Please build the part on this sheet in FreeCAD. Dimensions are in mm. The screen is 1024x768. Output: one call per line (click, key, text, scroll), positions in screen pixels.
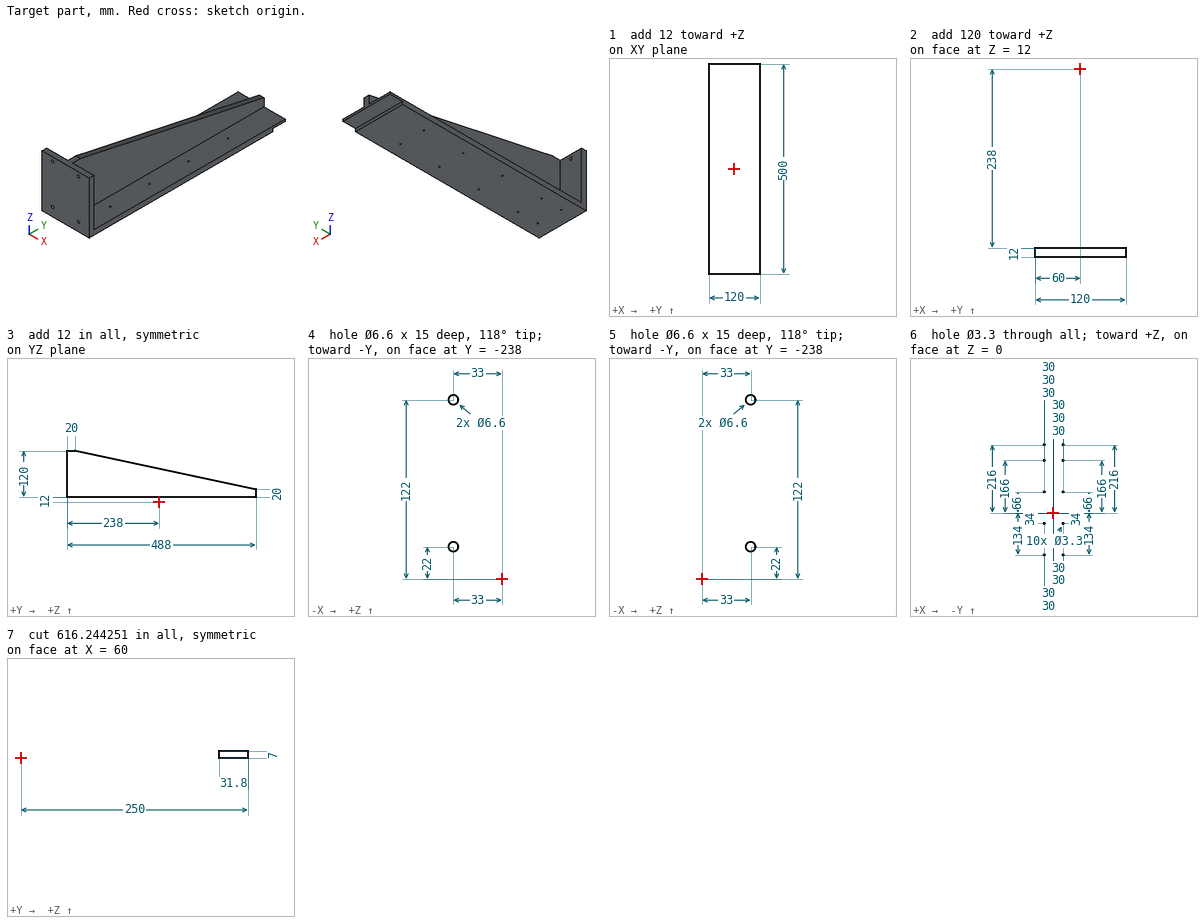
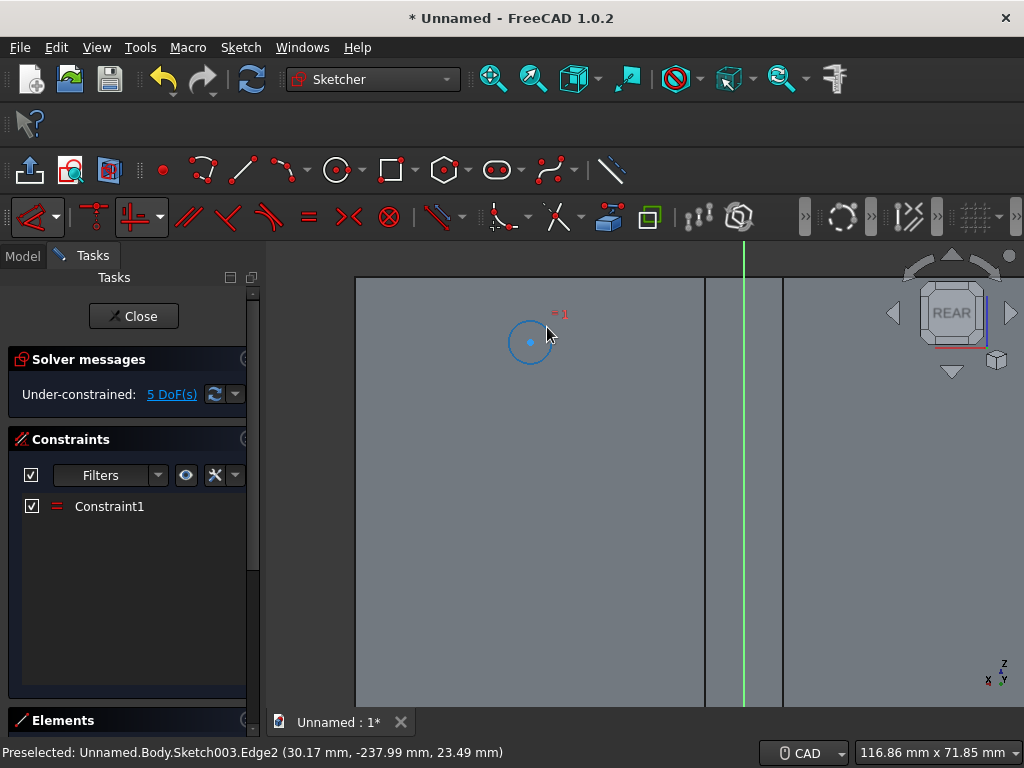
click(545, 327)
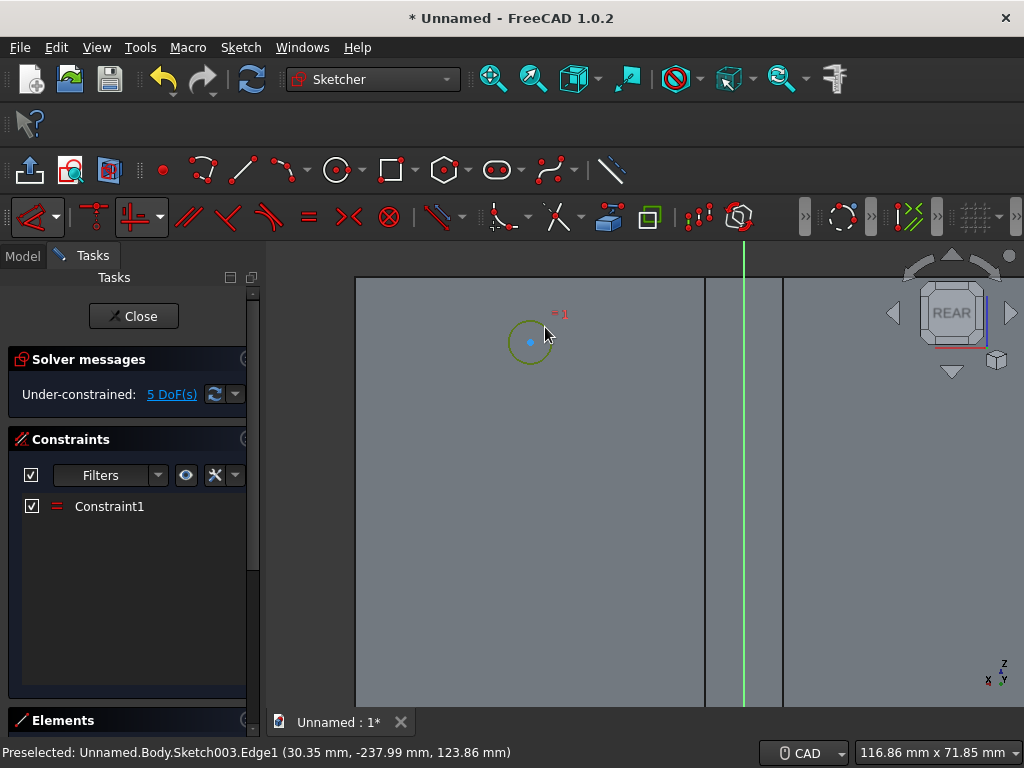
key(k)
key(o)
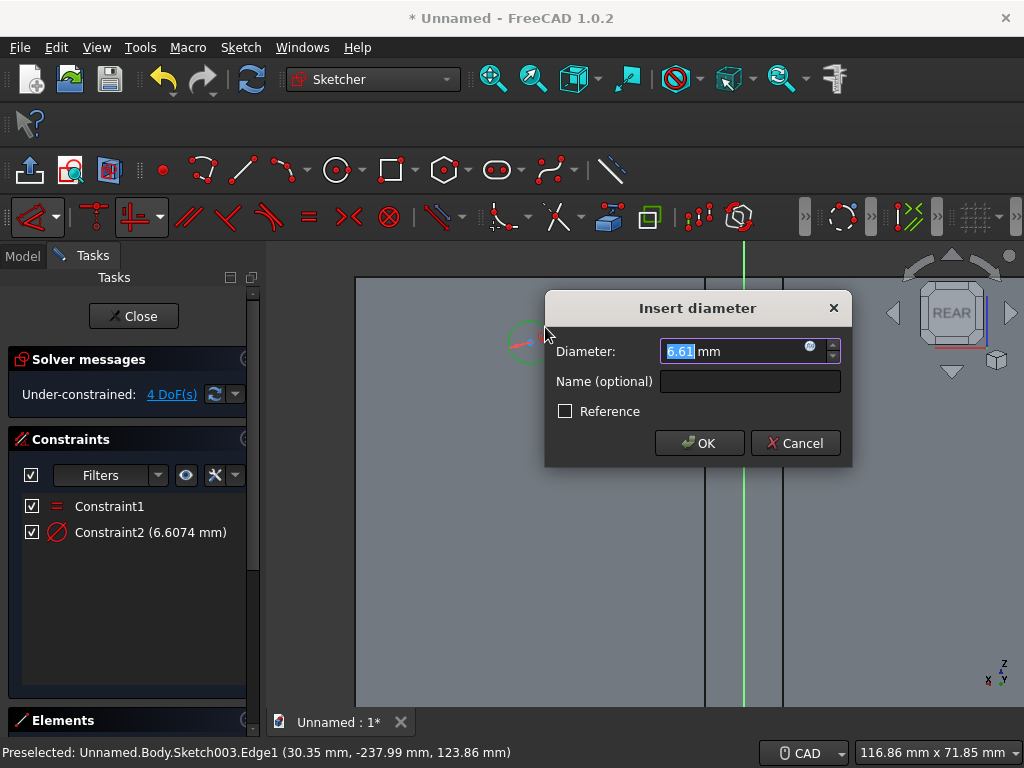
text(6.6)
key(Return)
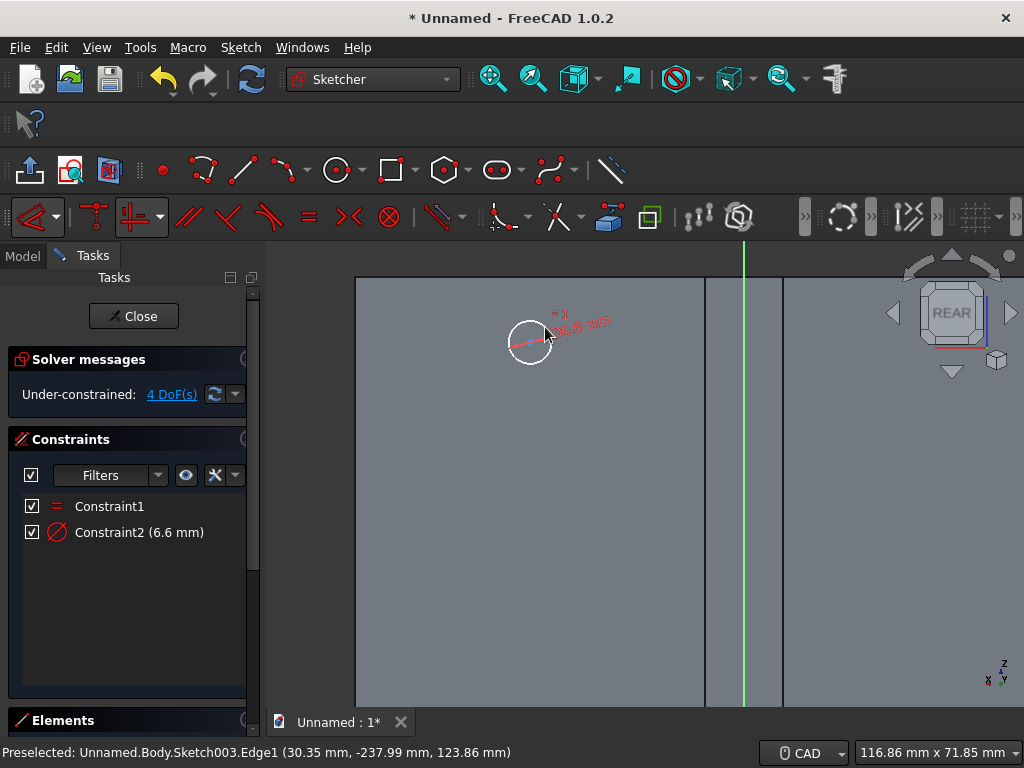
click(530, 342)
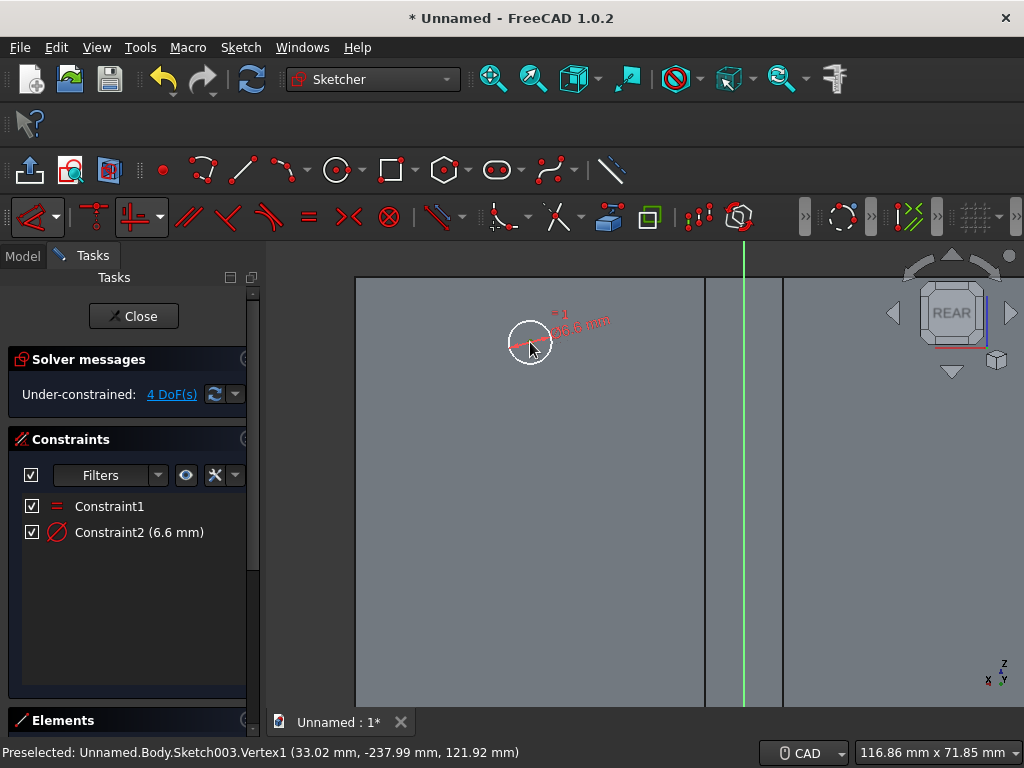
key(l)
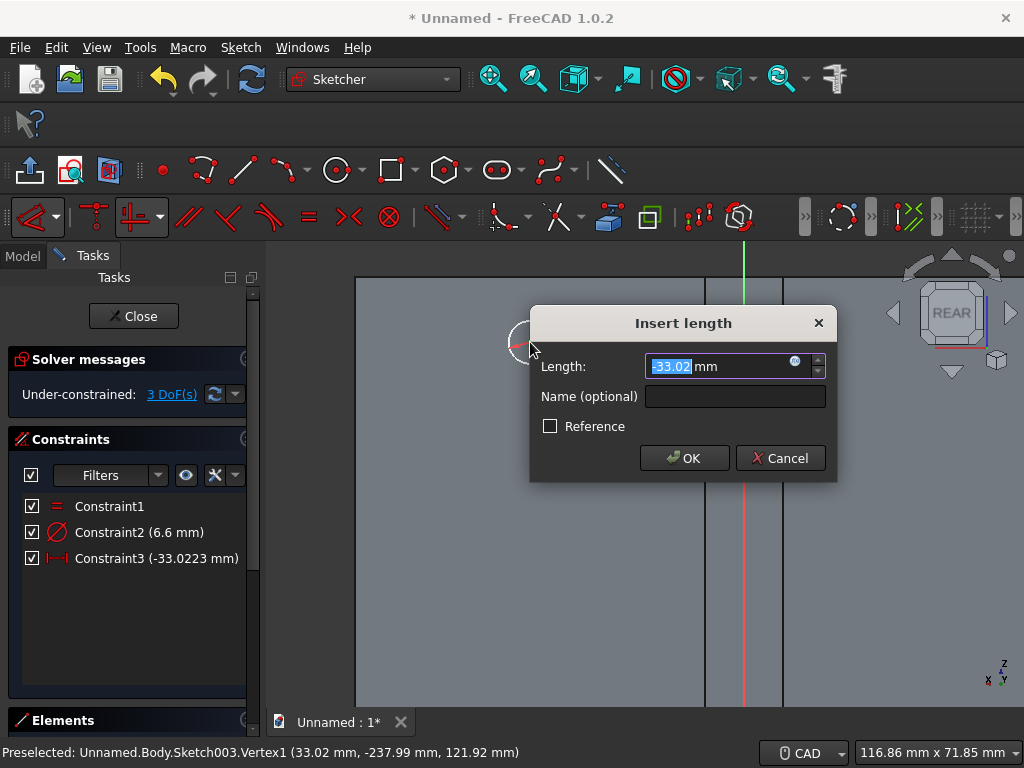
text(-33)
key(Return)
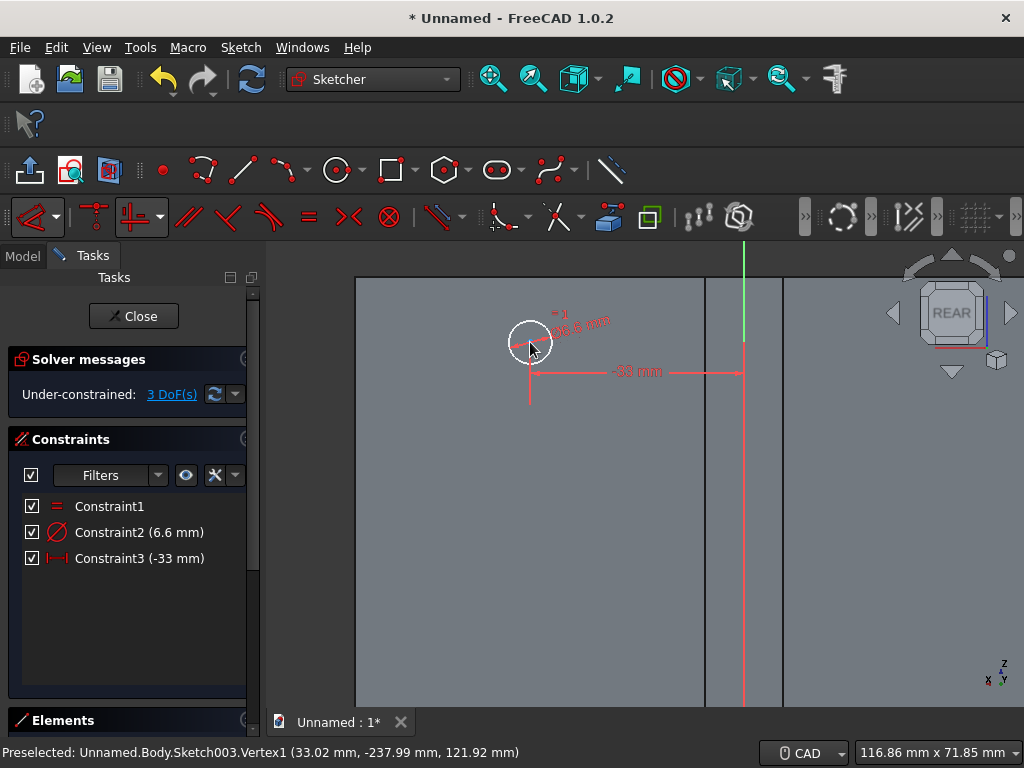
scroll(547, 327, down, 5)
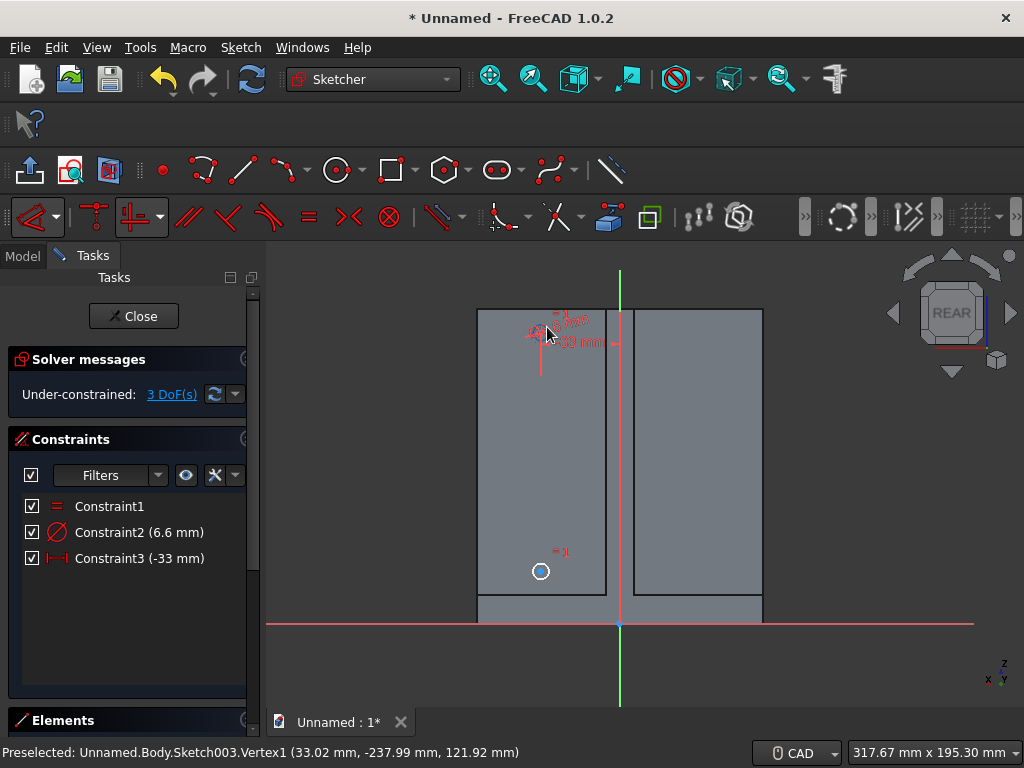
click(541, 571)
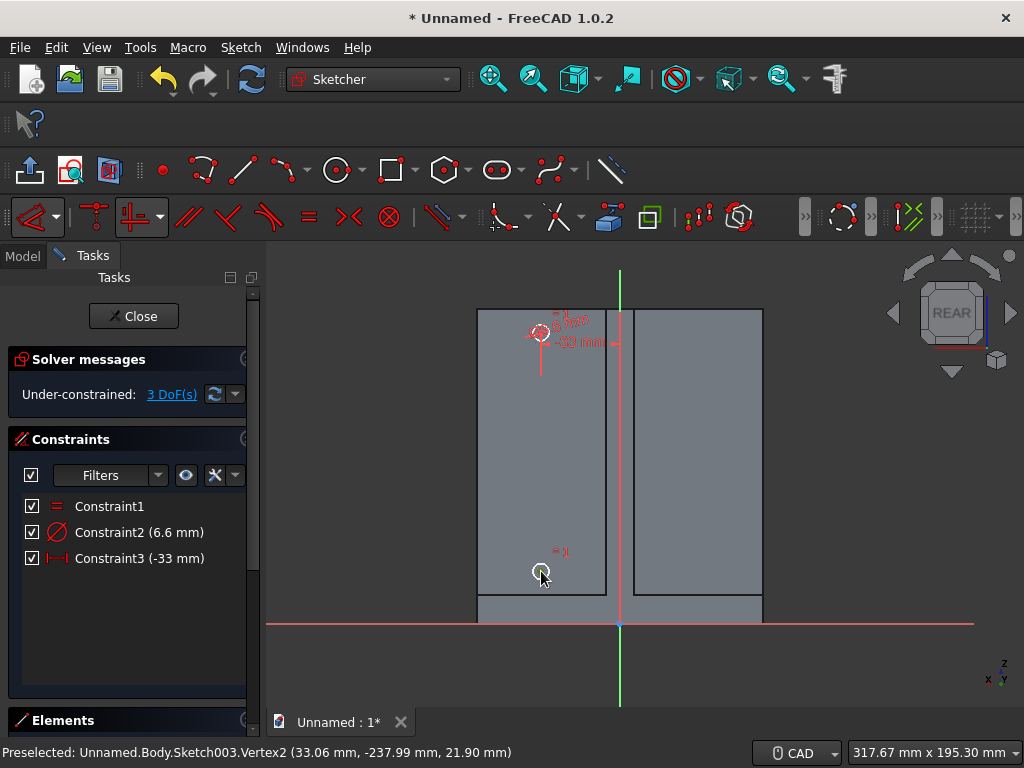
key(l)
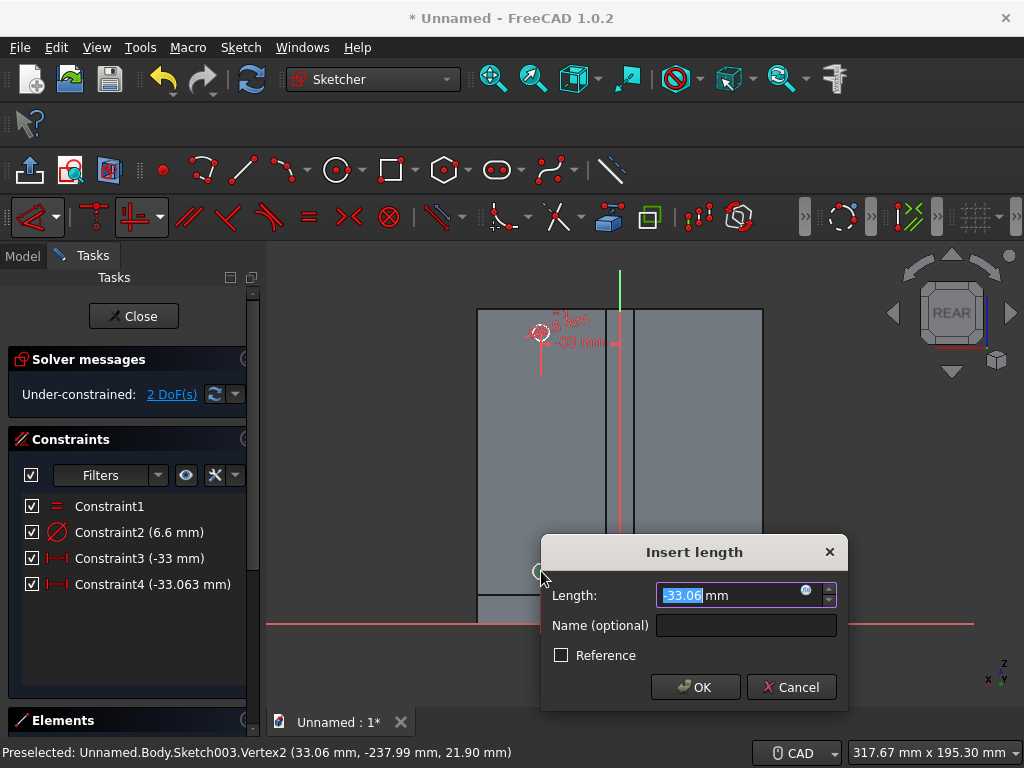
text(-33)
key(Return)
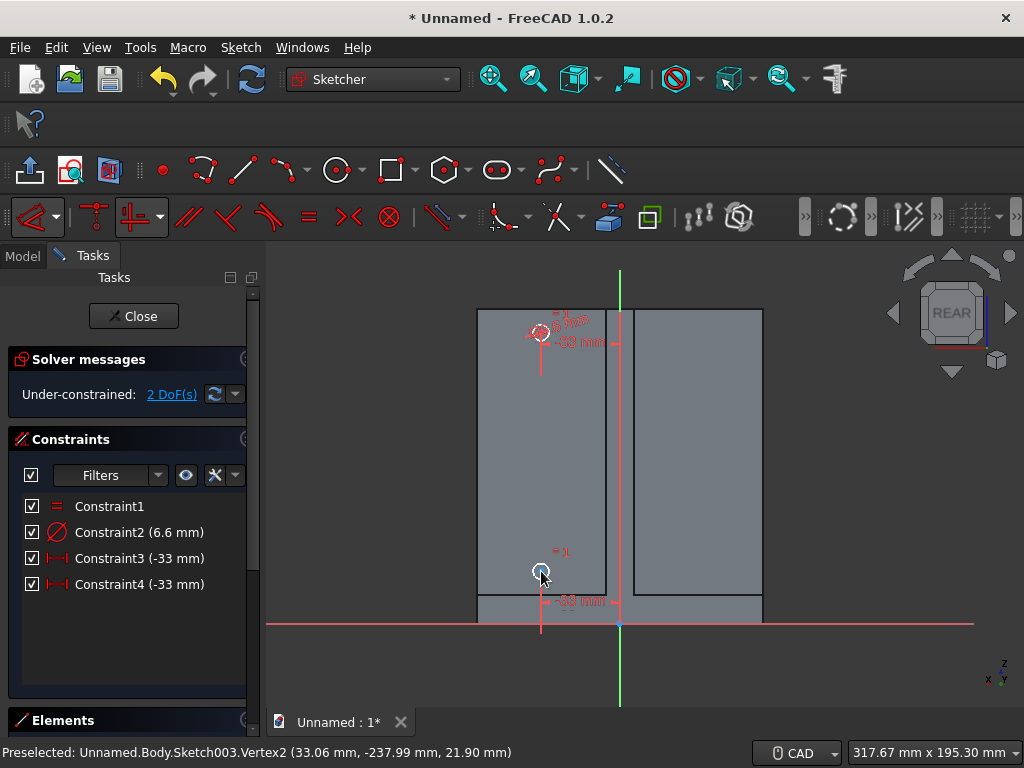
click(541, 571)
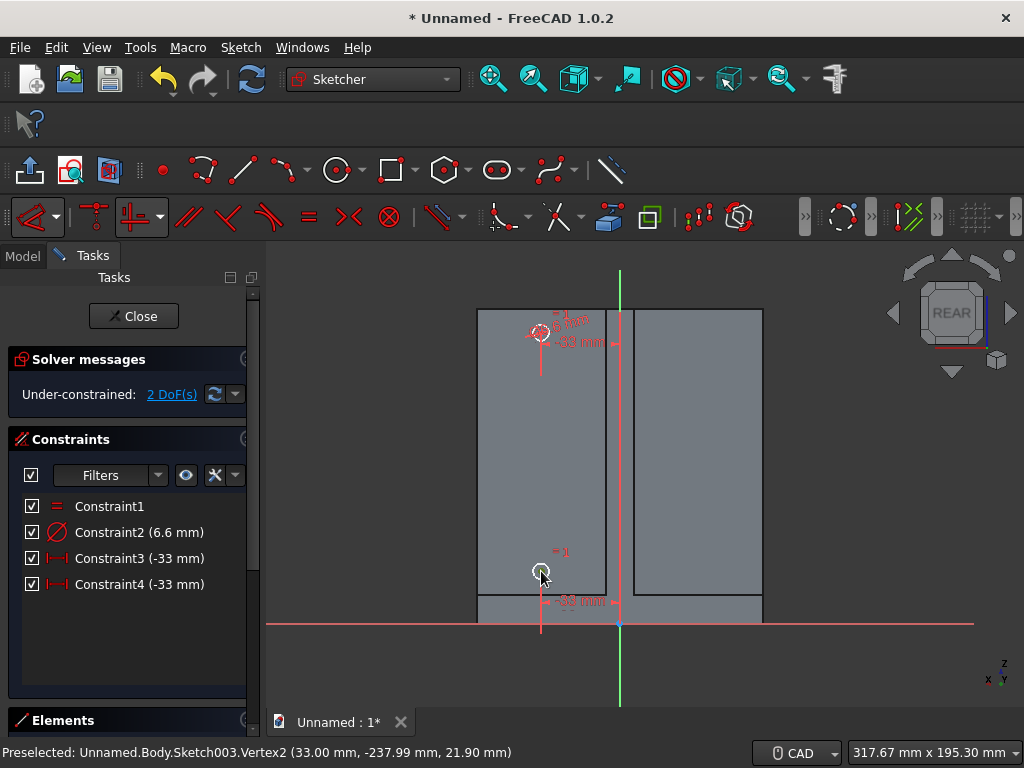
key(i)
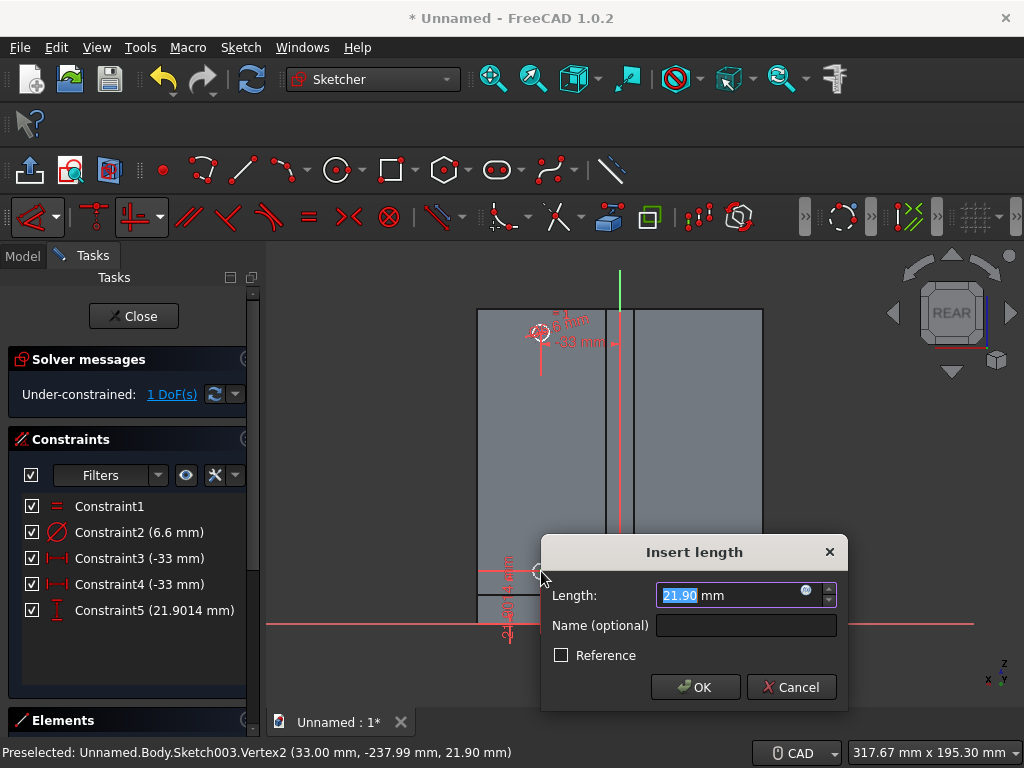
text(22)
key(Return)